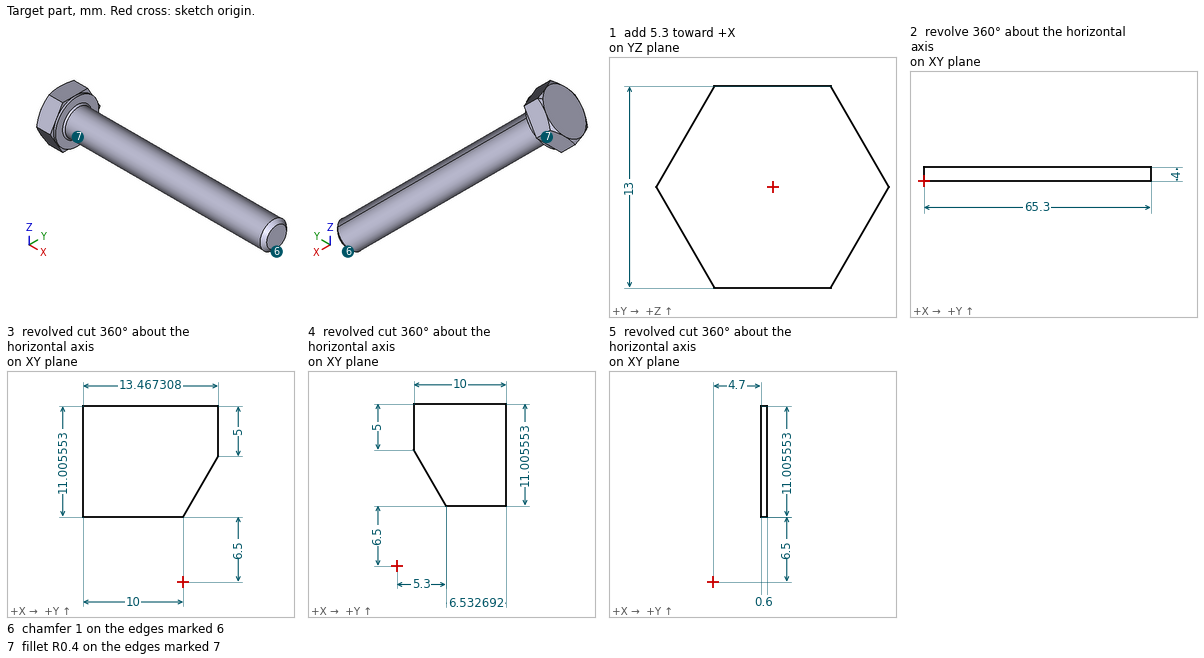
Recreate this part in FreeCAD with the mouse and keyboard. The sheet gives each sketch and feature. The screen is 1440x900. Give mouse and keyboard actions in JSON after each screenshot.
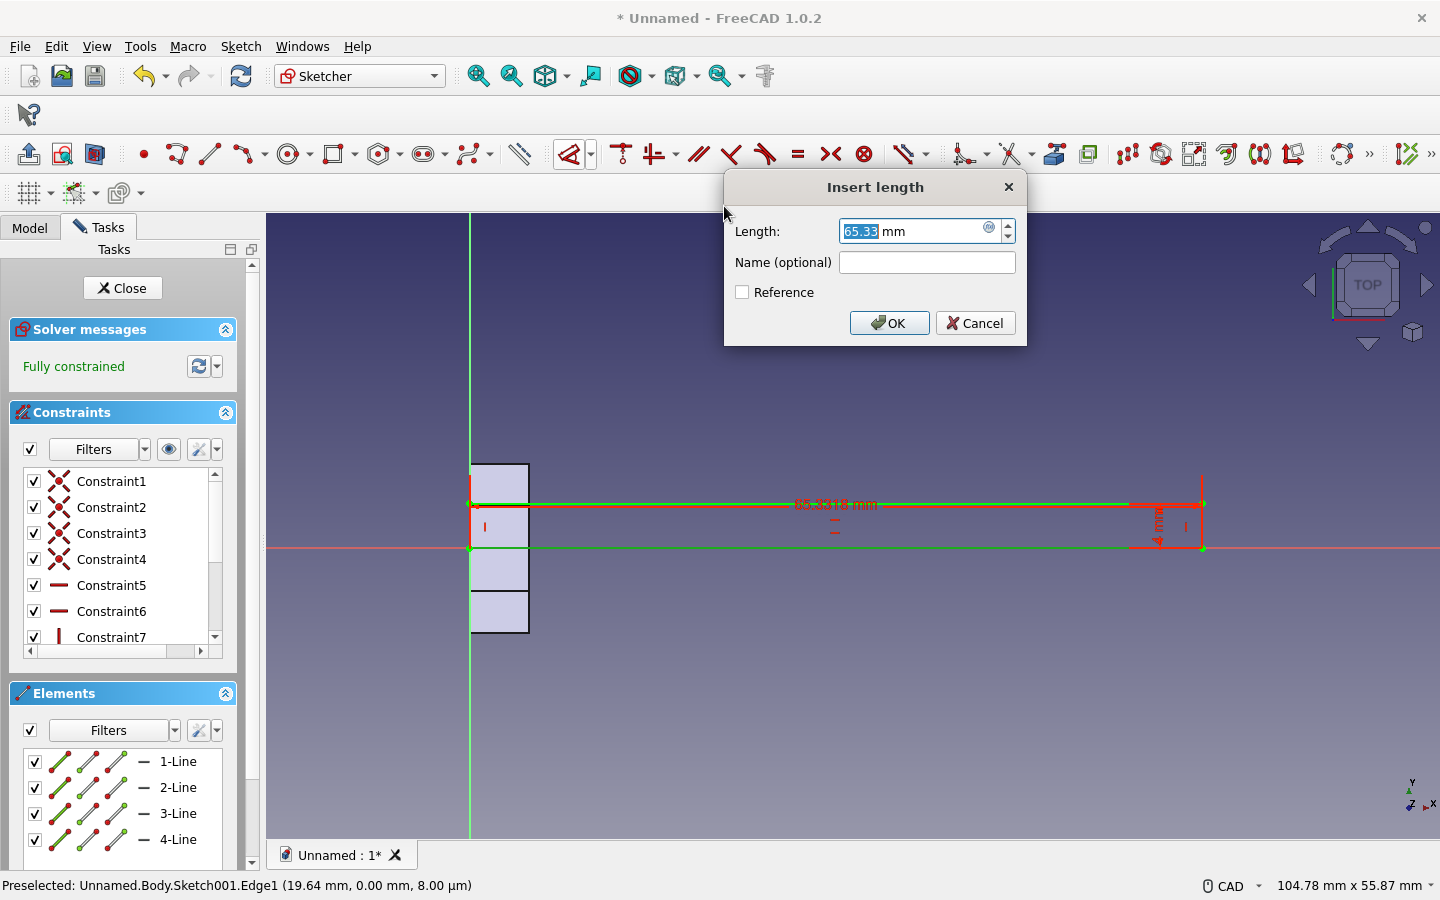
{"action": "type", "text": "65.3"}
{"action": "key", "text": "Return"}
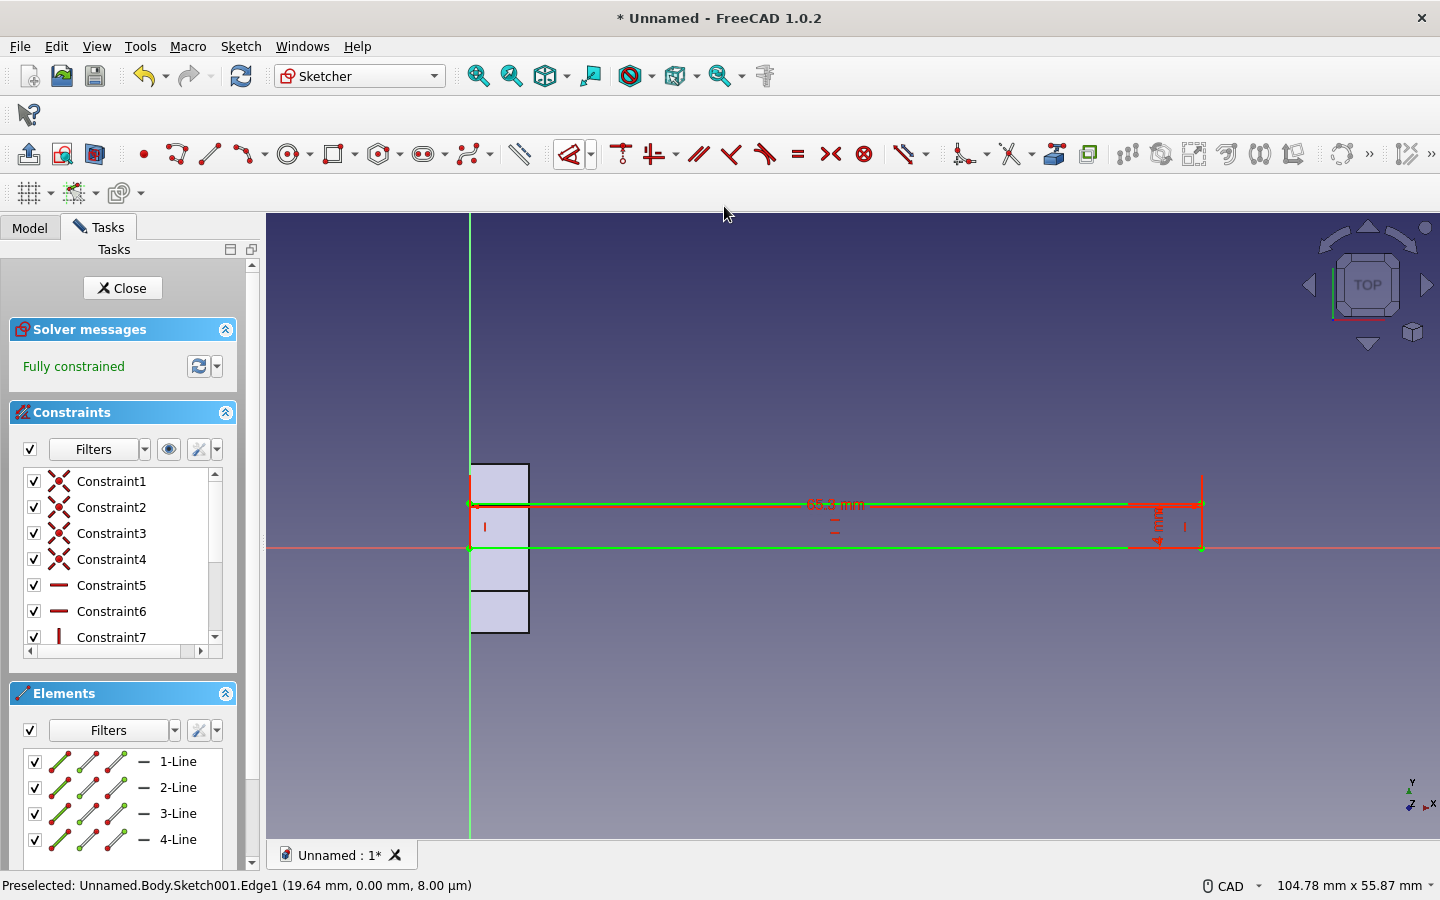
{"action": "left_click", "coordinate": [123, 288]}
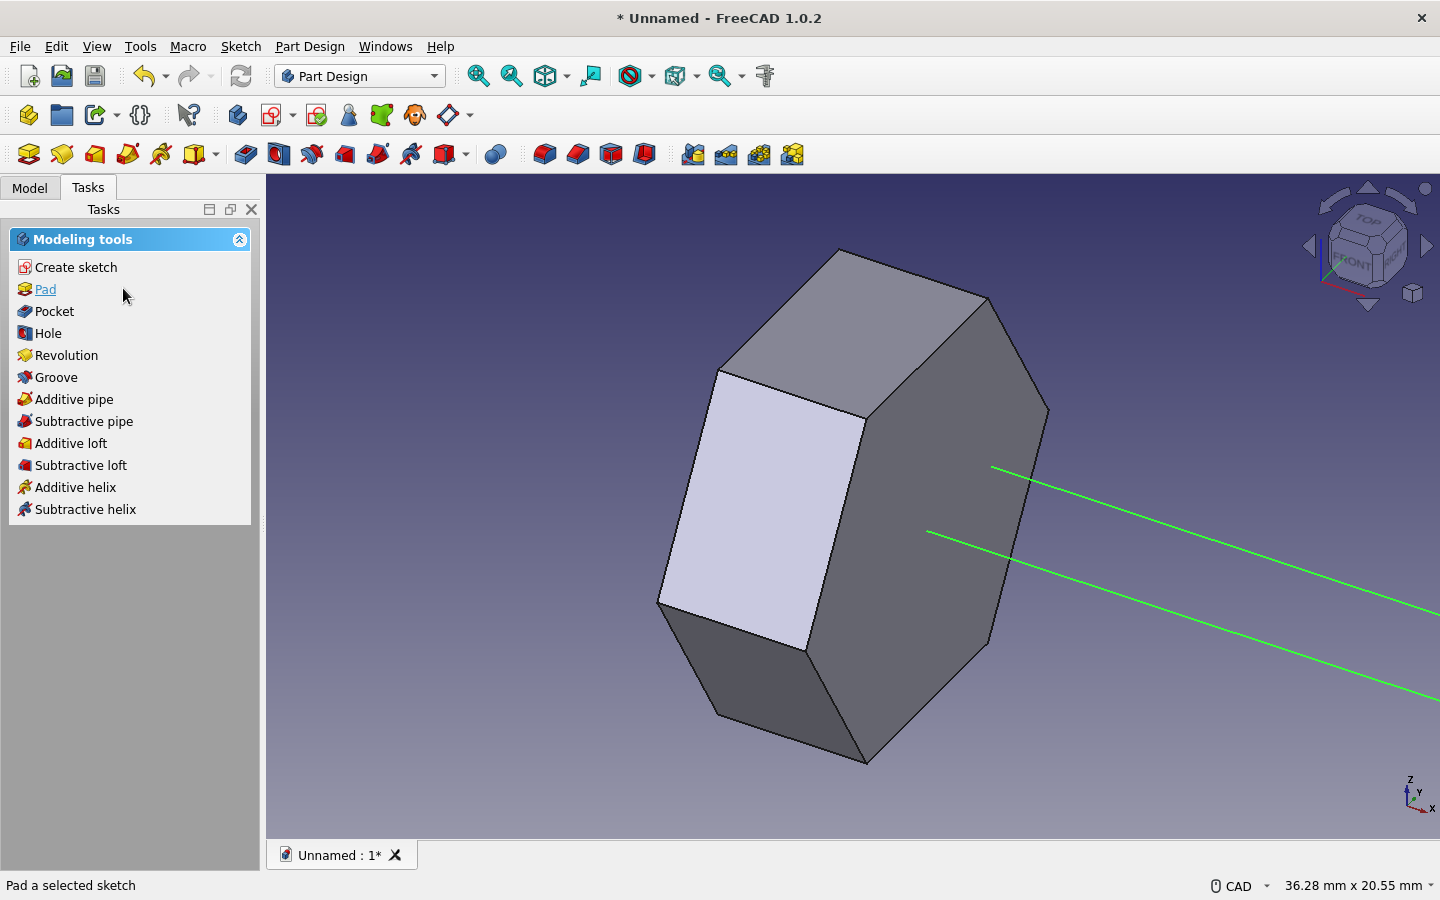
{"action": "left_click", "coordinate": [62, 154]}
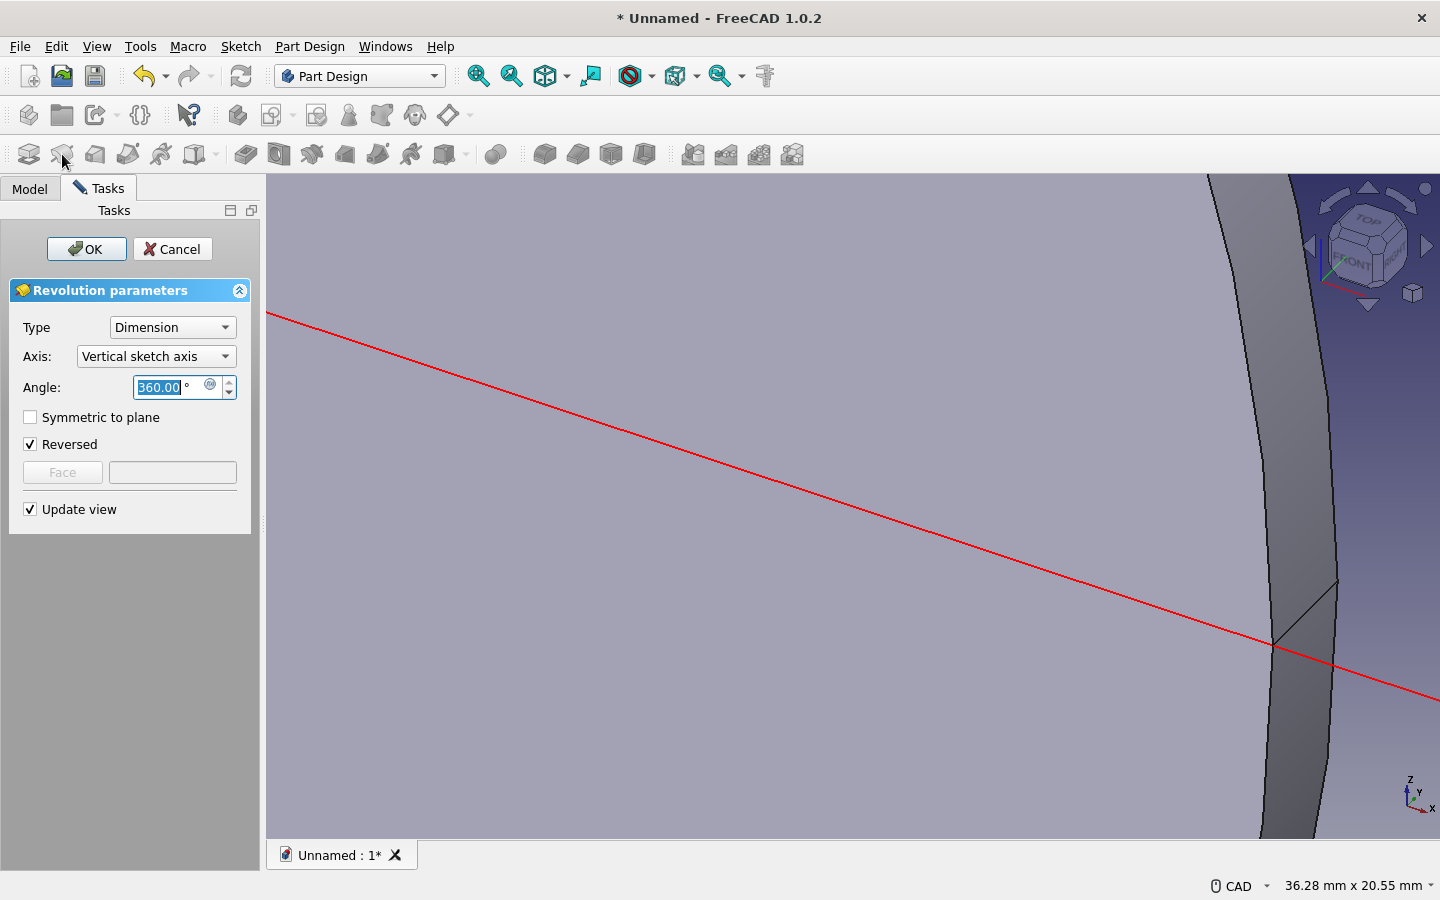
{"action": "left_click", "coordinate": [157, 356]}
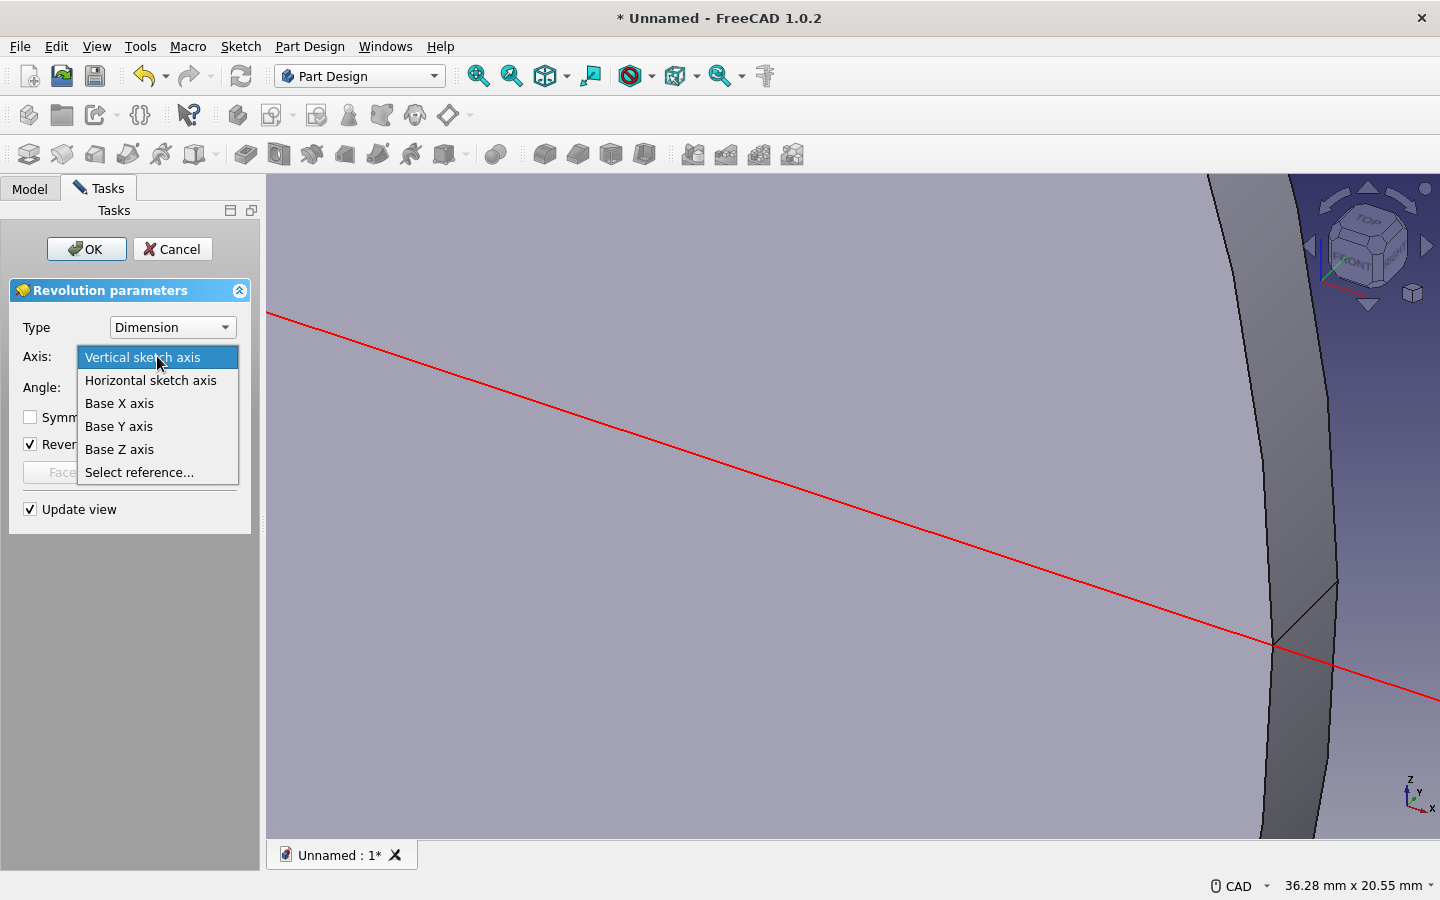
{"action": "left_click", "coordinate": [156, 380]}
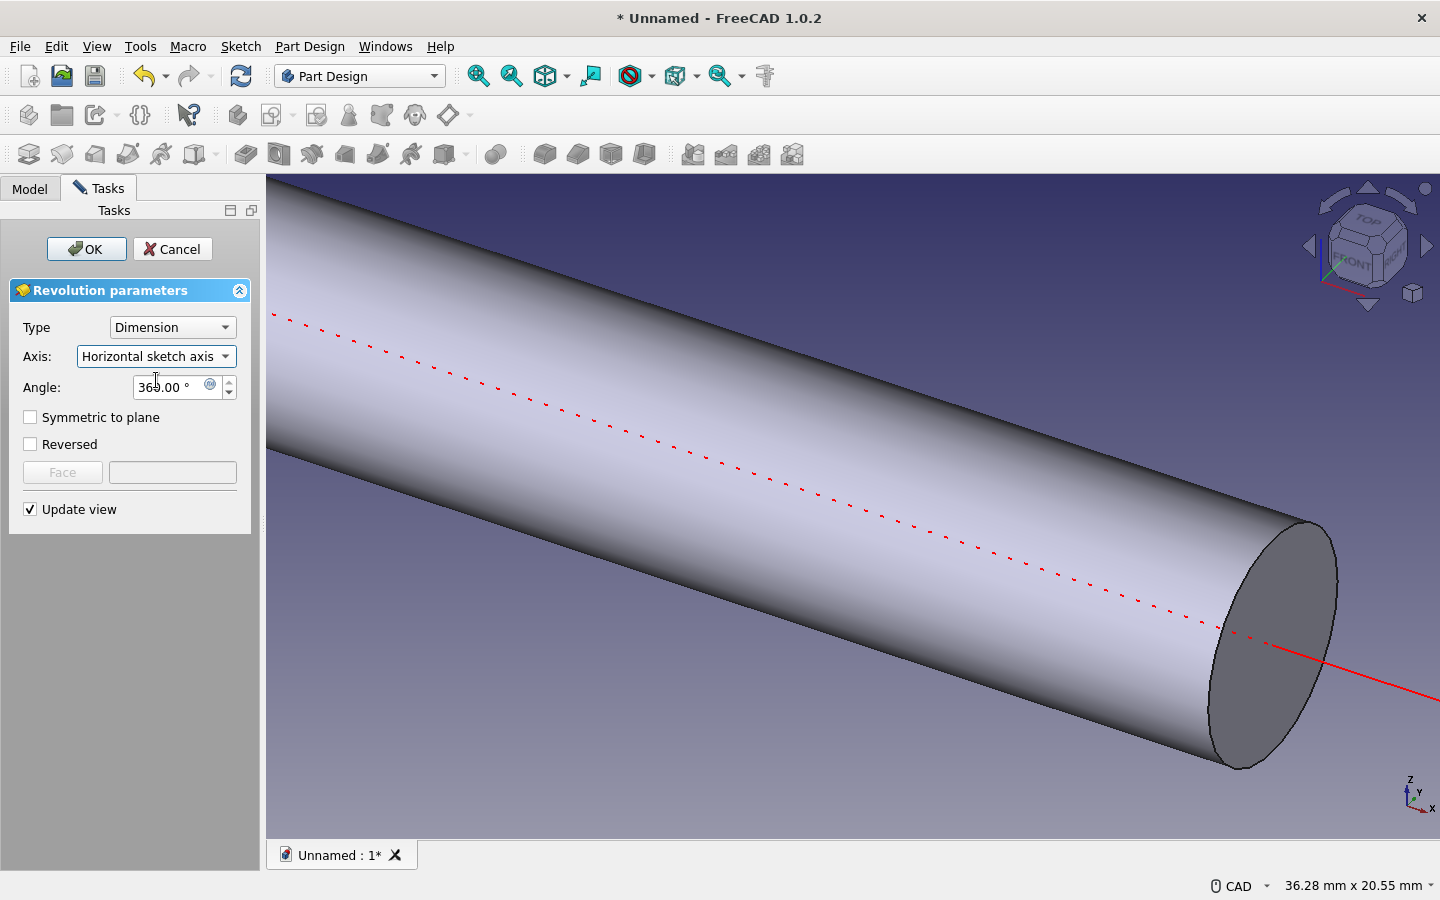
{"action": "left_click", "coordinate": [87, 249]}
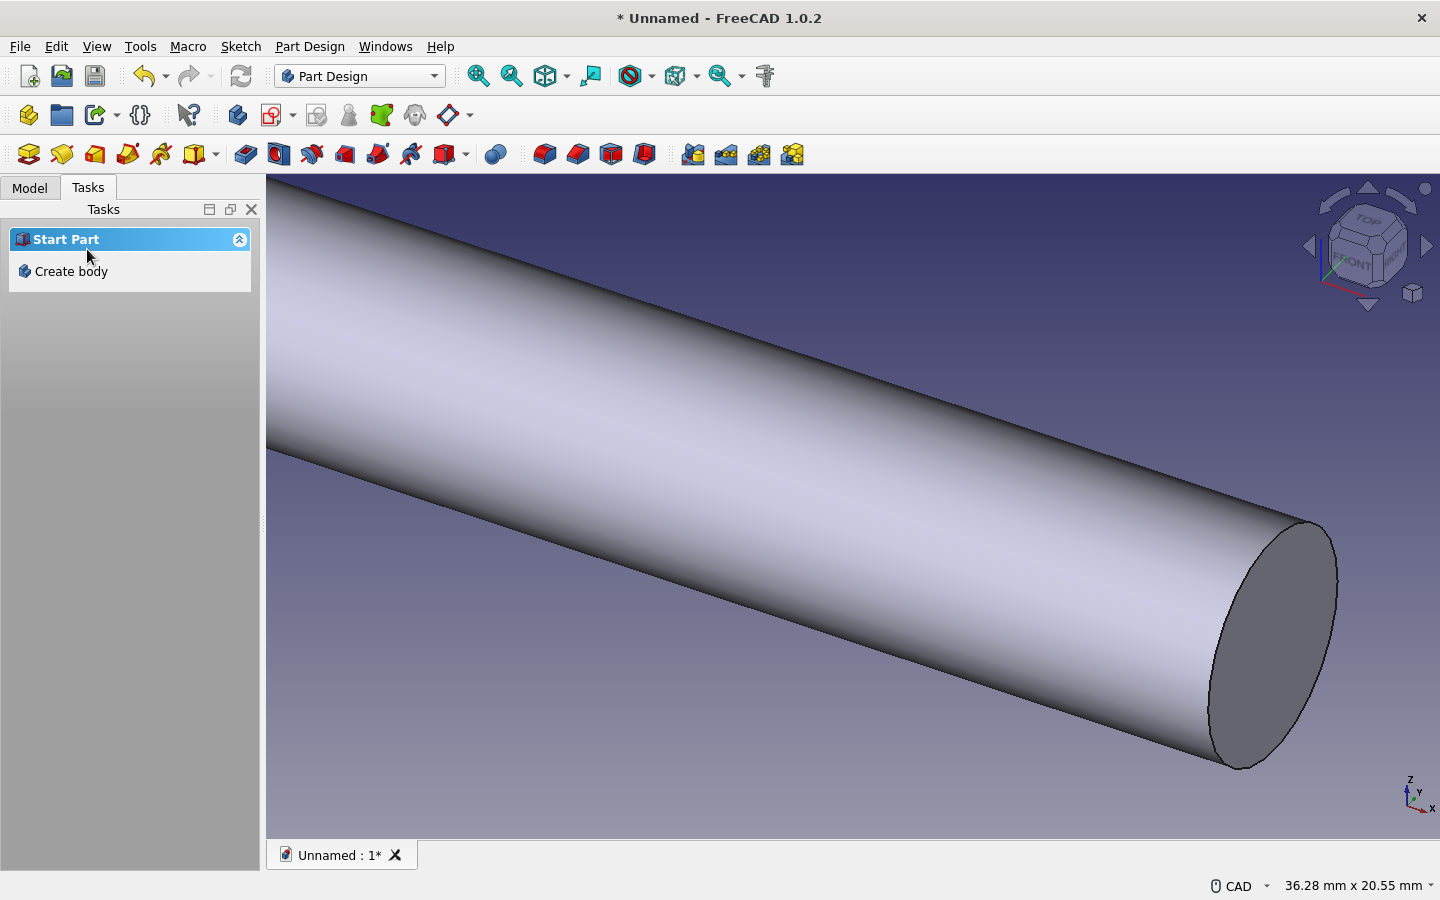
{"action": "left_click", "coordinate": [479, 76]}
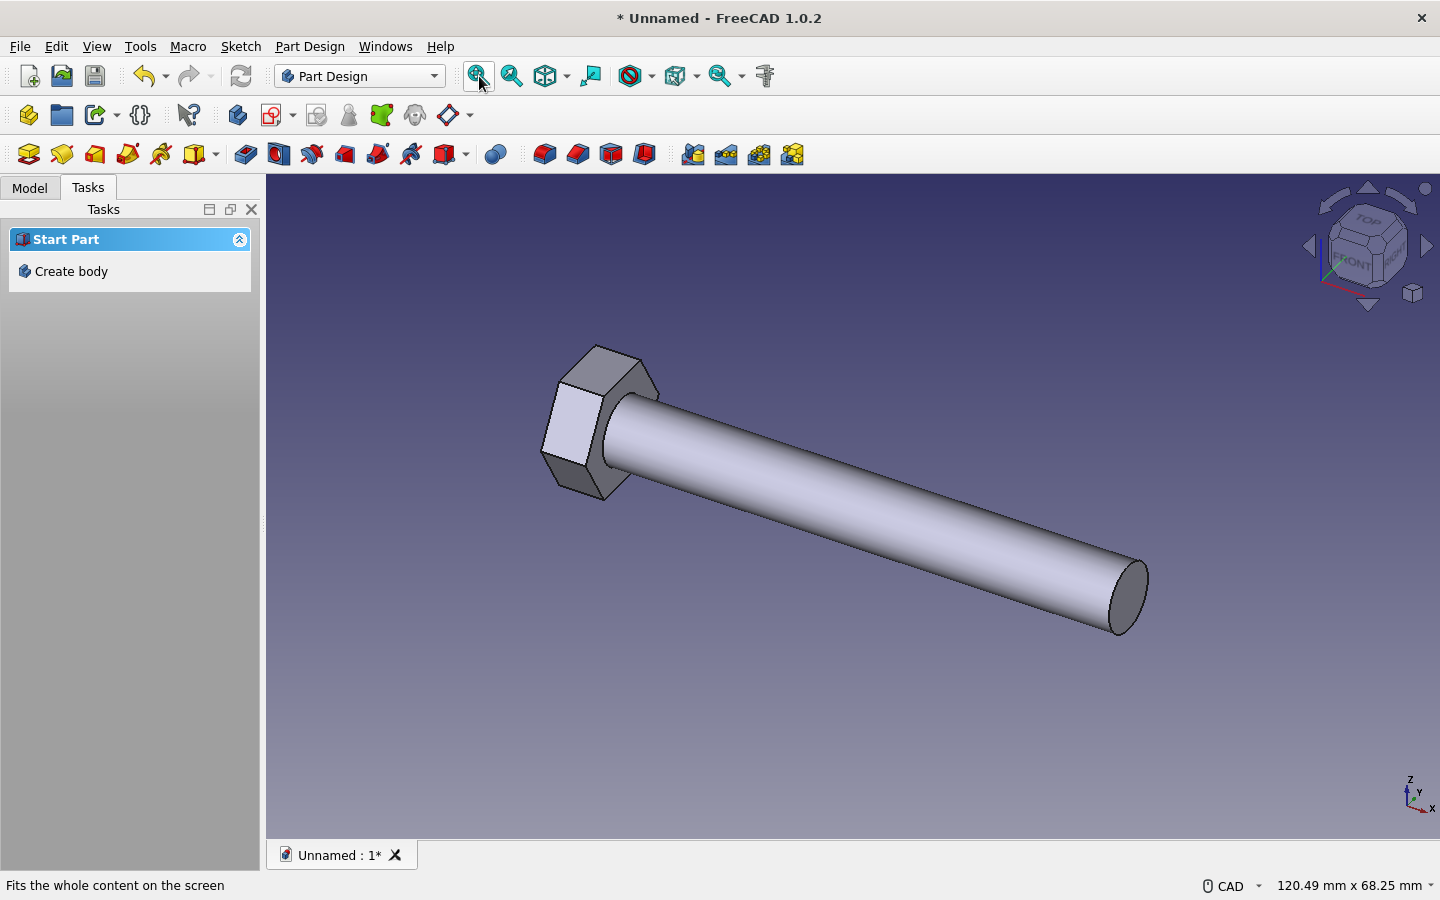
{"action": "left_click", "coordinate": [270, 116]}